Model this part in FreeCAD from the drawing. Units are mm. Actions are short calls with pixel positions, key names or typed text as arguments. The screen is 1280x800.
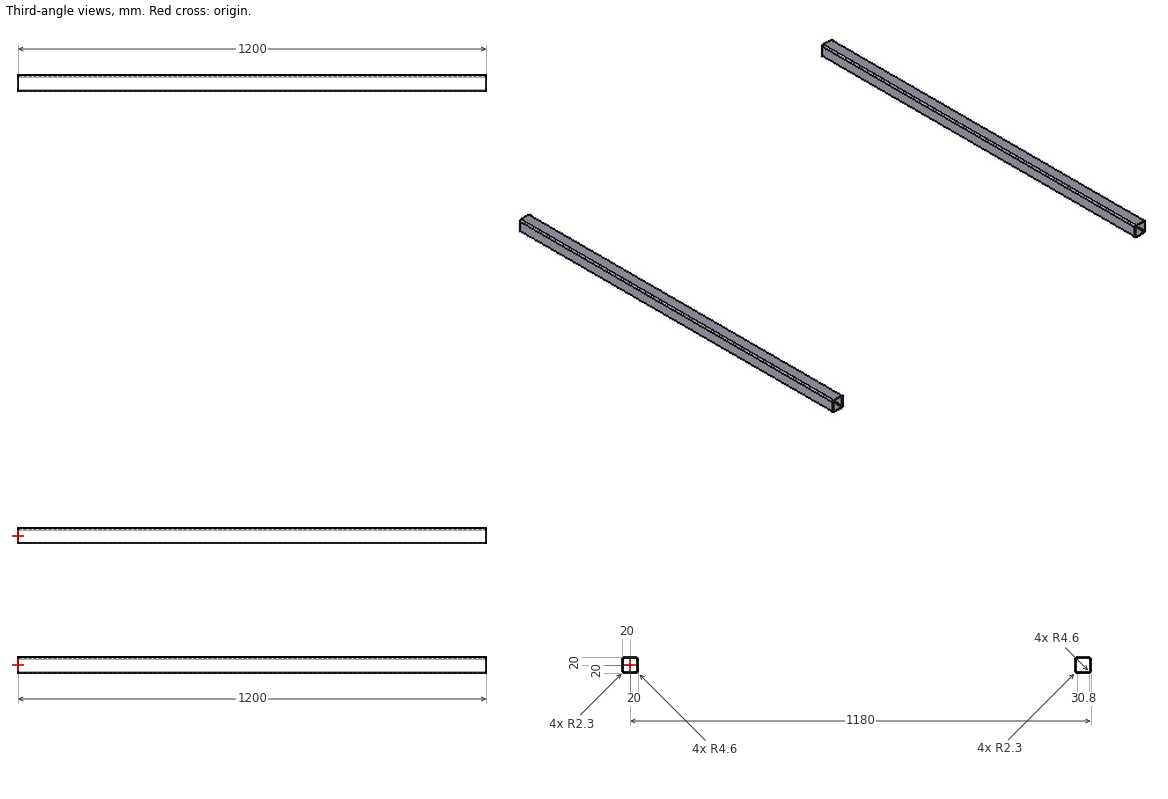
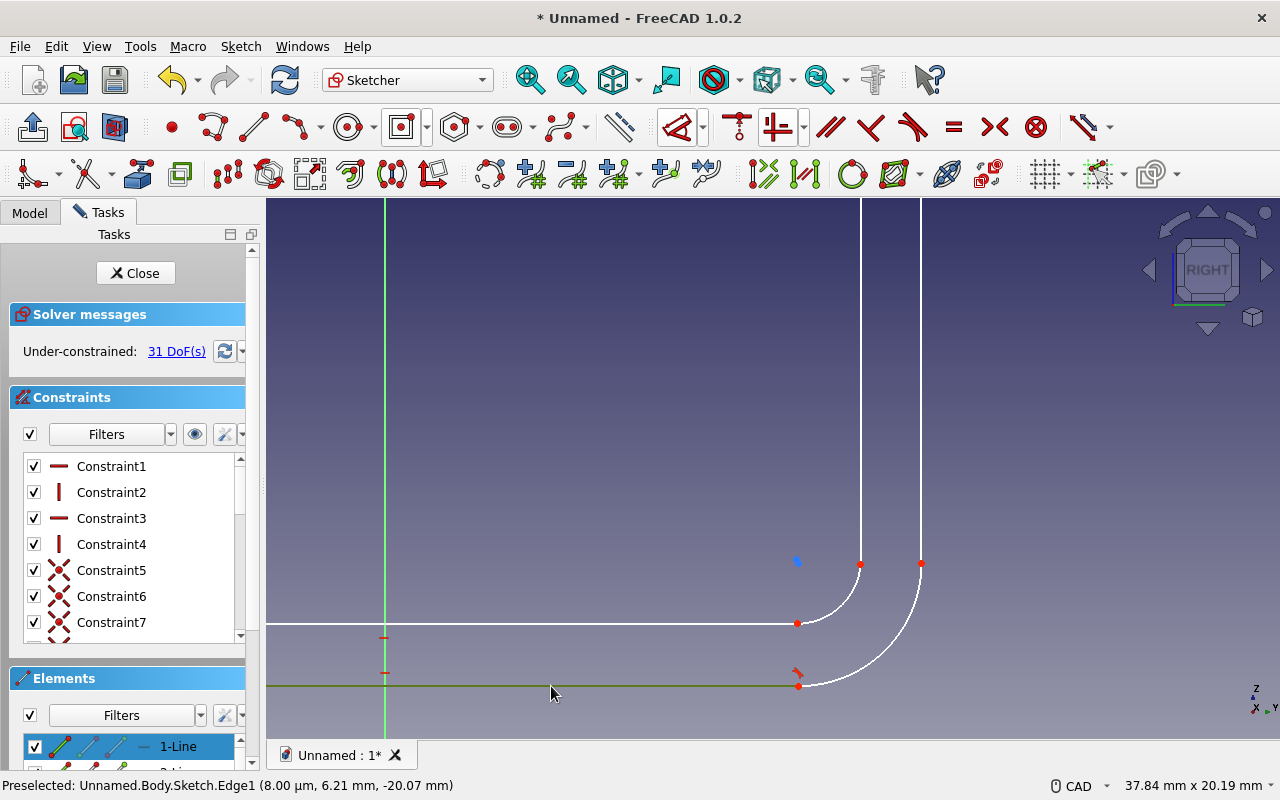
scroll(842, 607, down, 6)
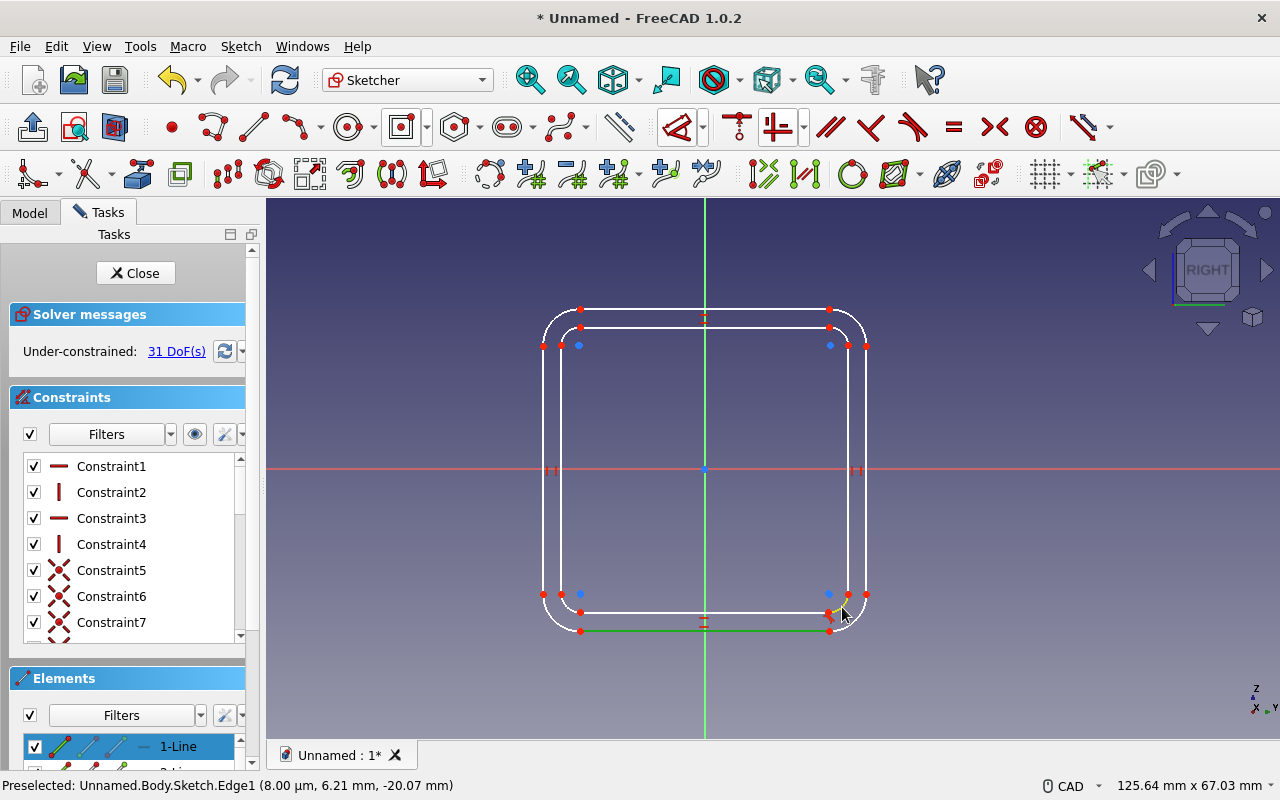
click(547, 611)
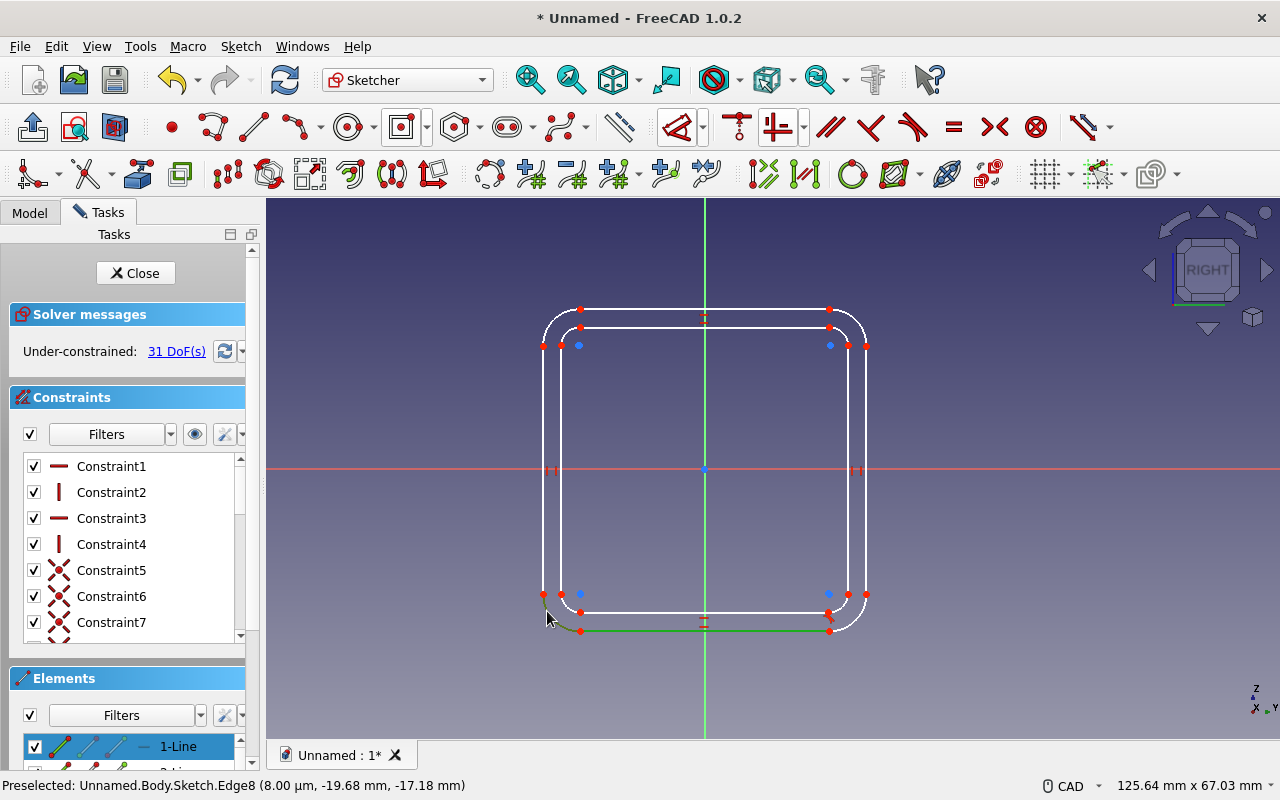
click(913, 128)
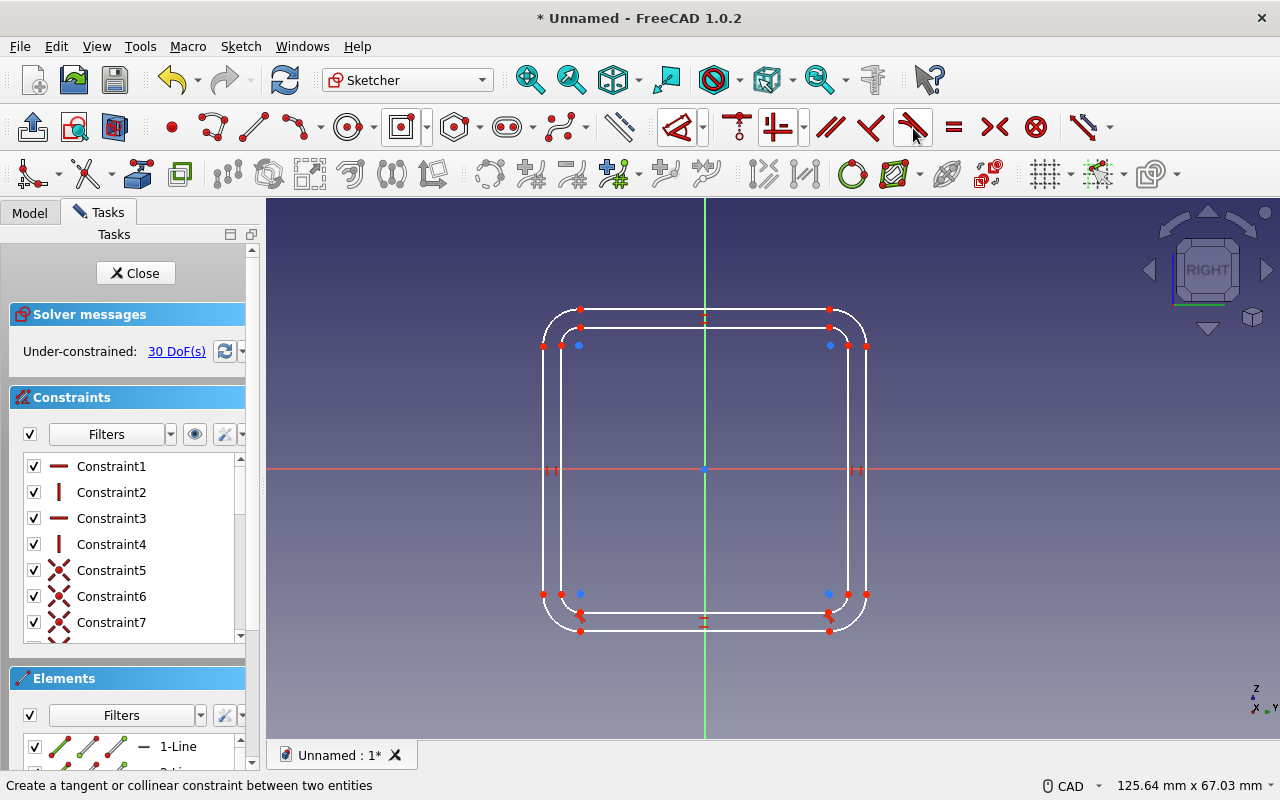
click(866, 520)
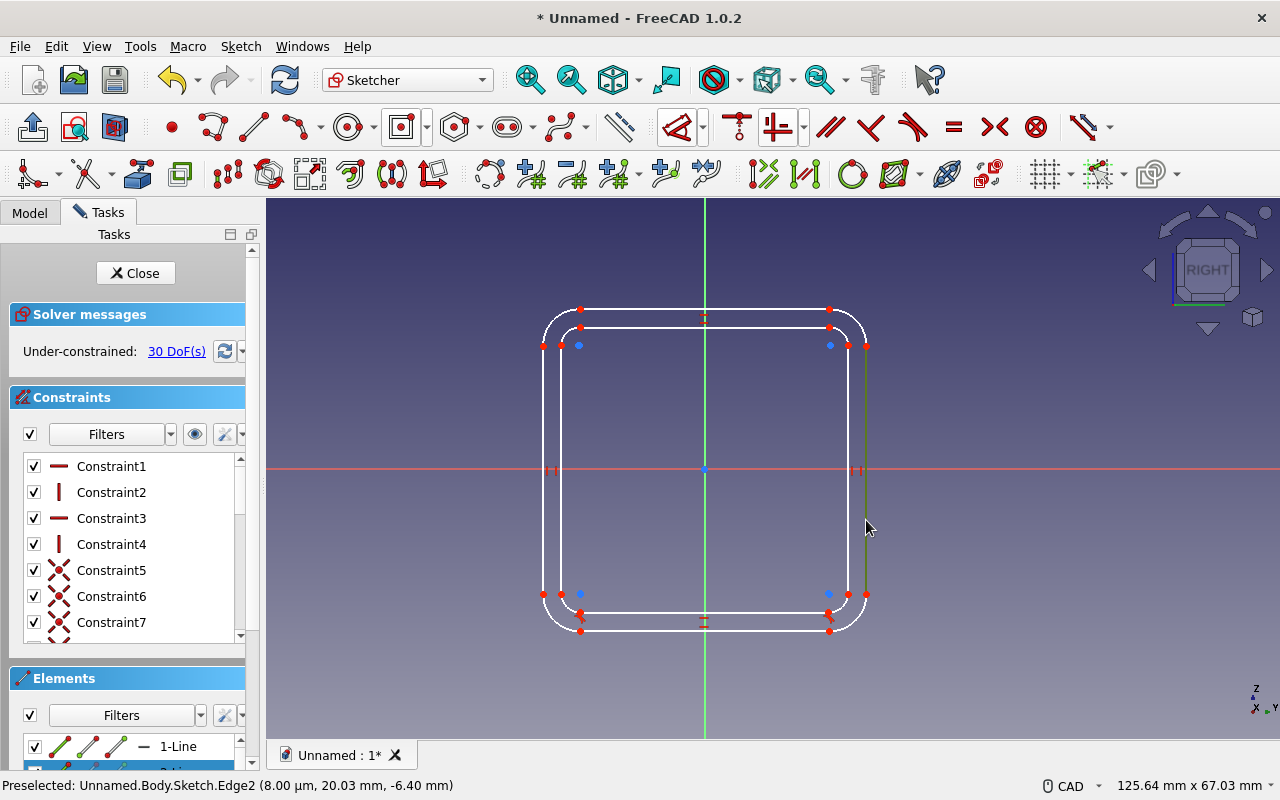
click(846, 627)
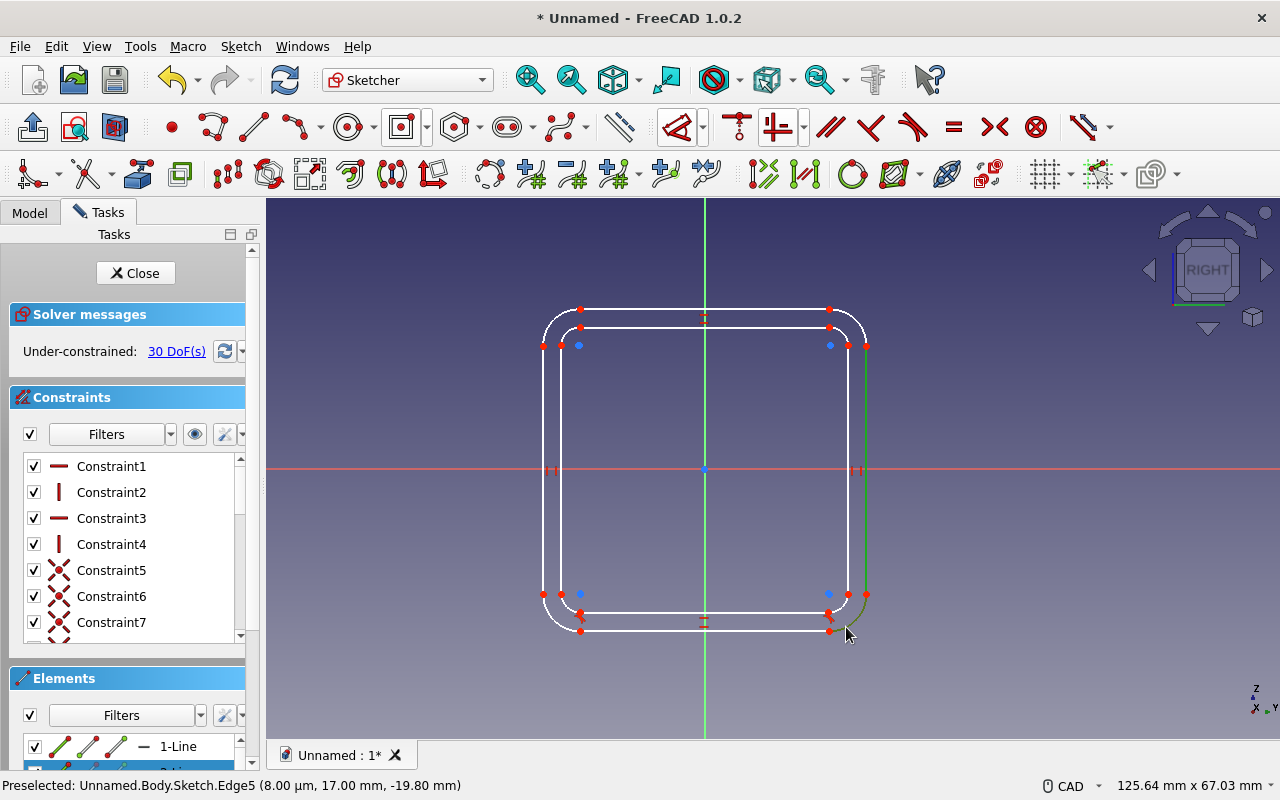
key(t)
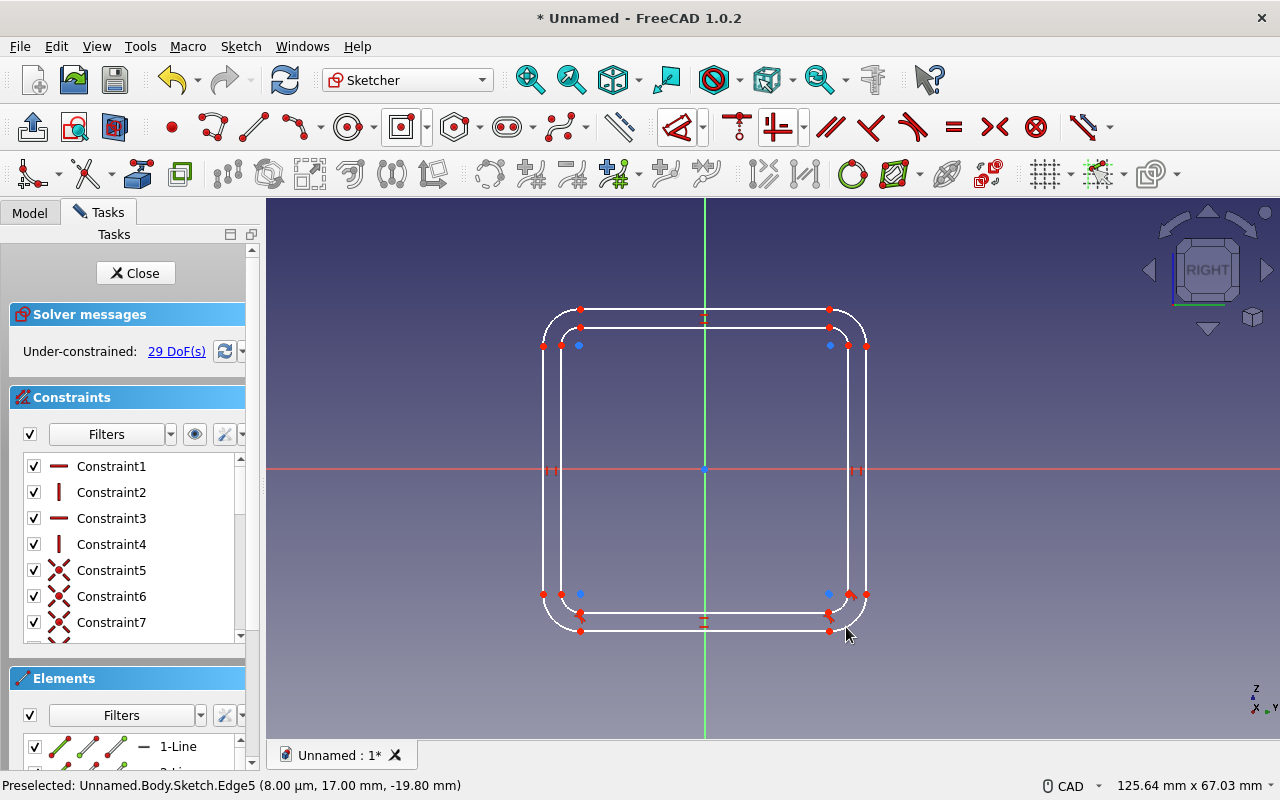
click(866, 520)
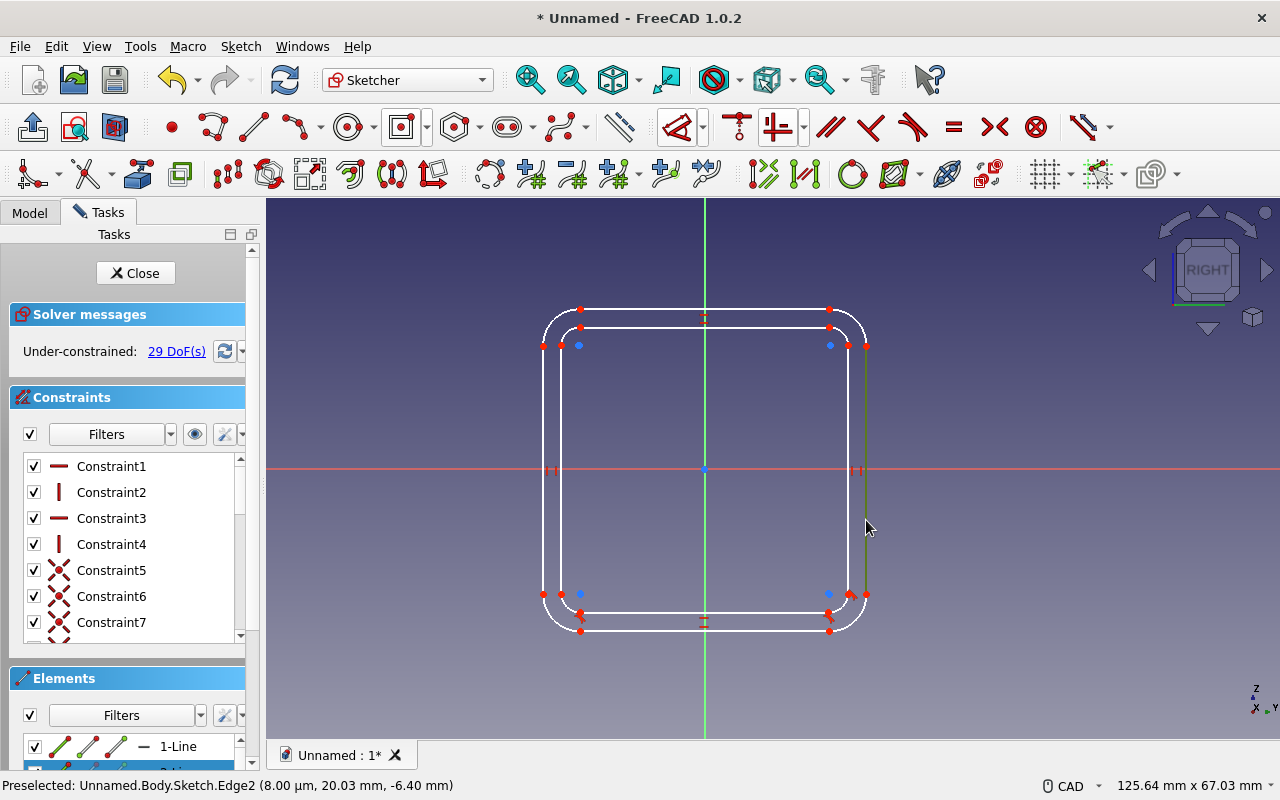
click(863, 329)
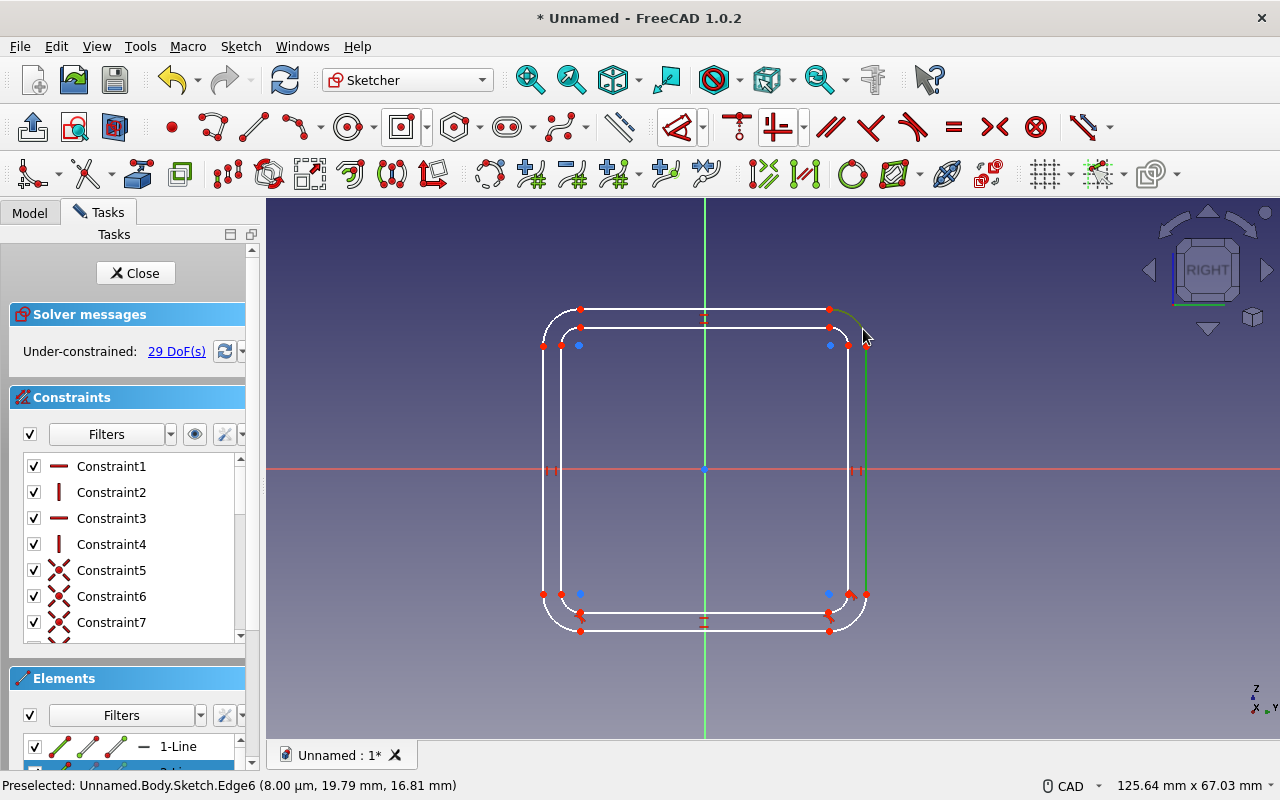
key(t)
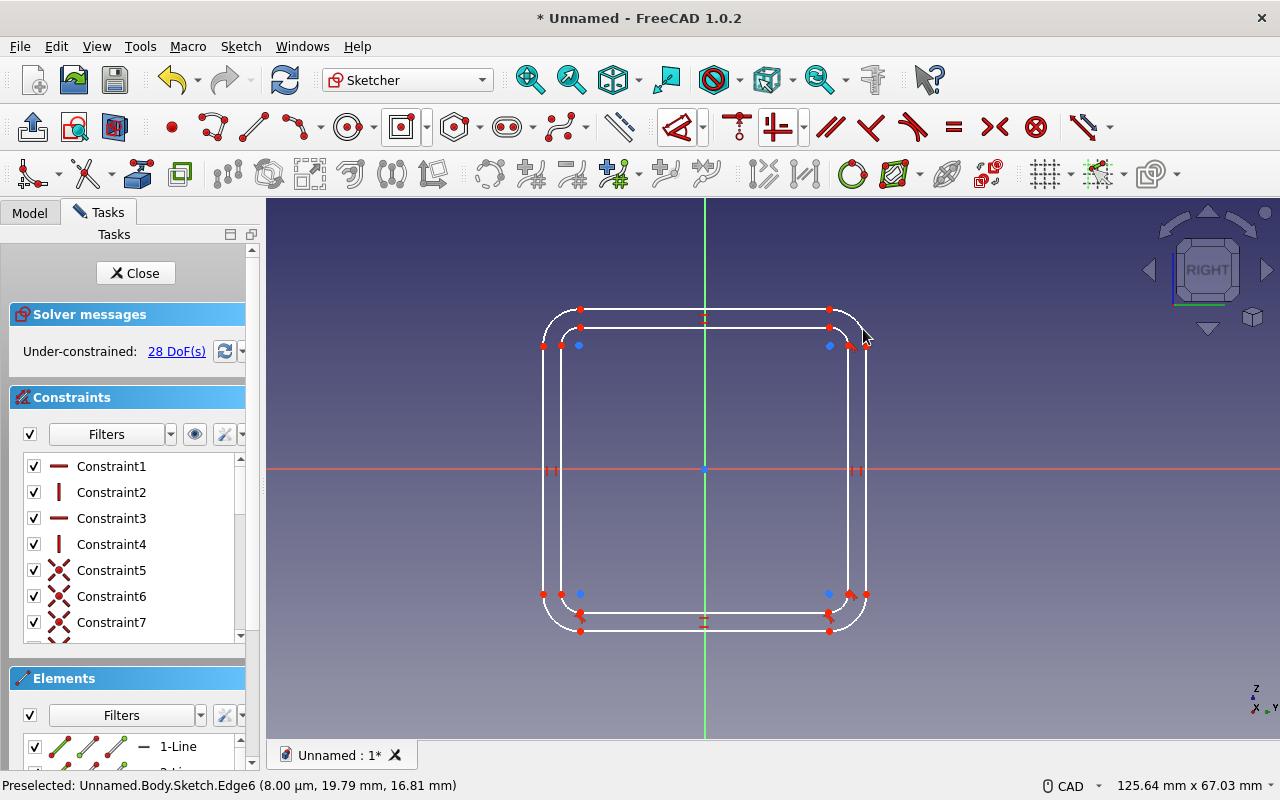
click(755, 309)